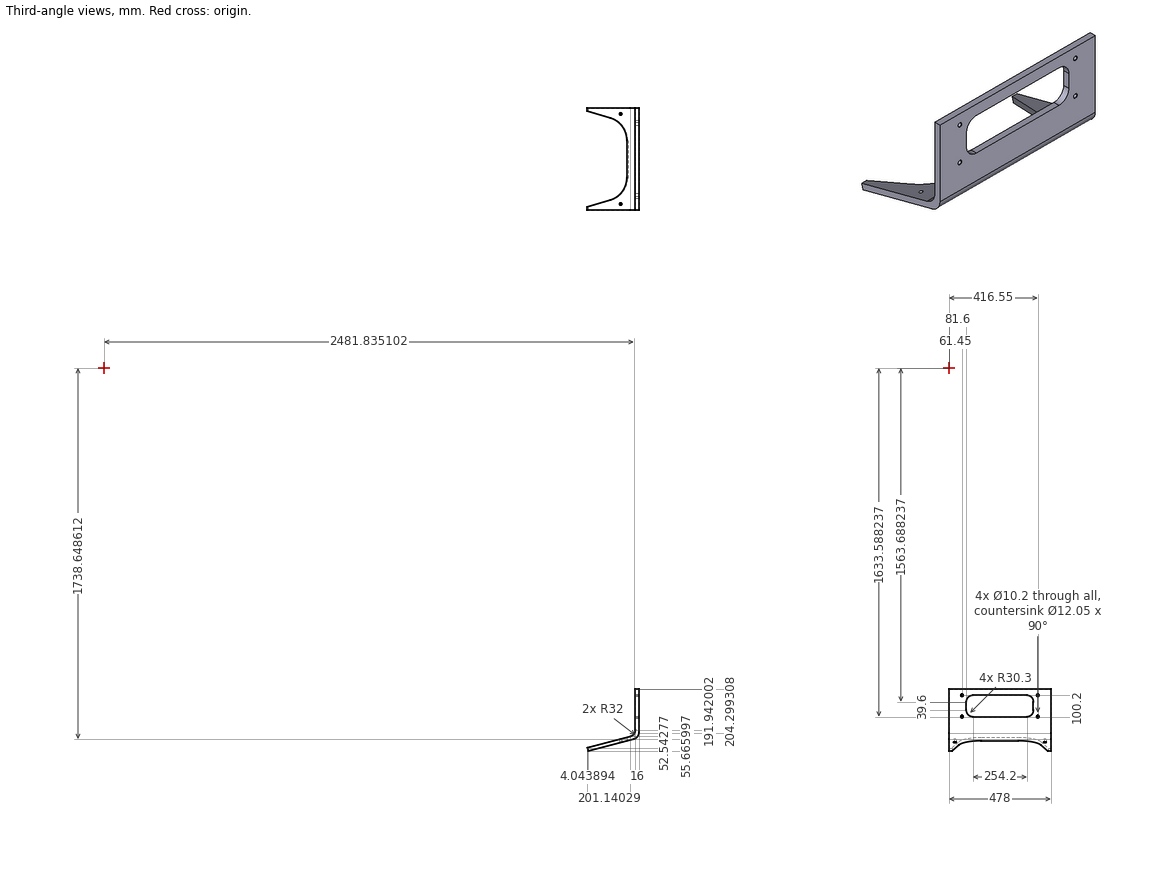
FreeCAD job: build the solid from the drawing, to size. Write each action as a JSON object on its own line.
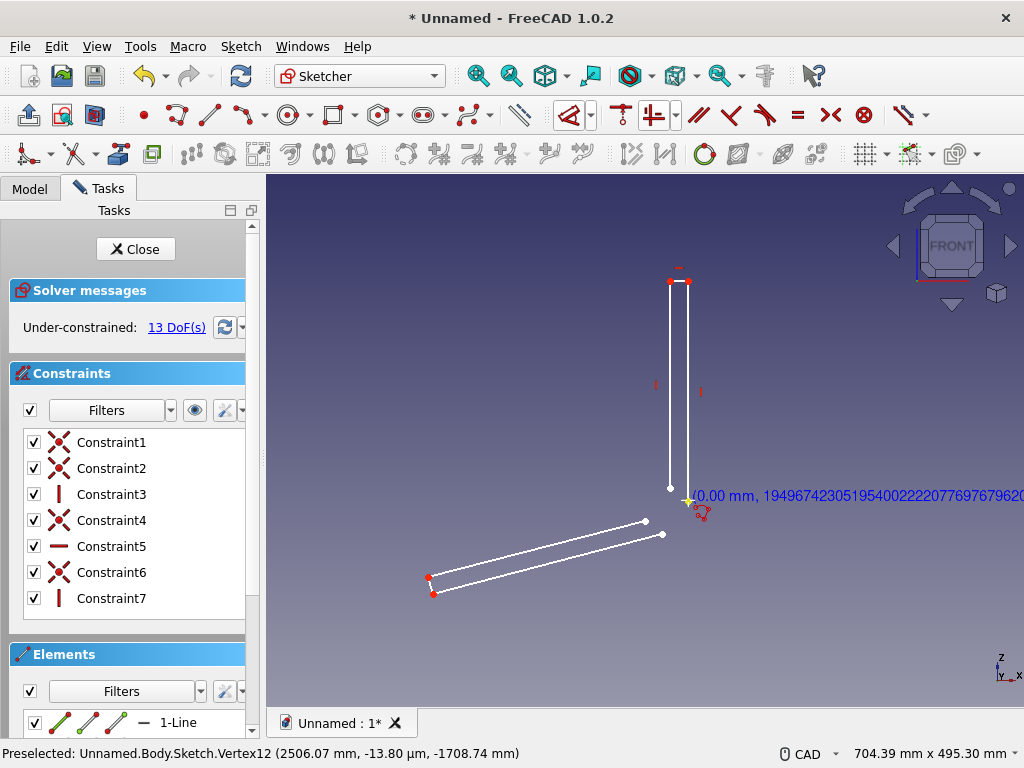
{"action": "left_click", "coordinate": [242, 116]}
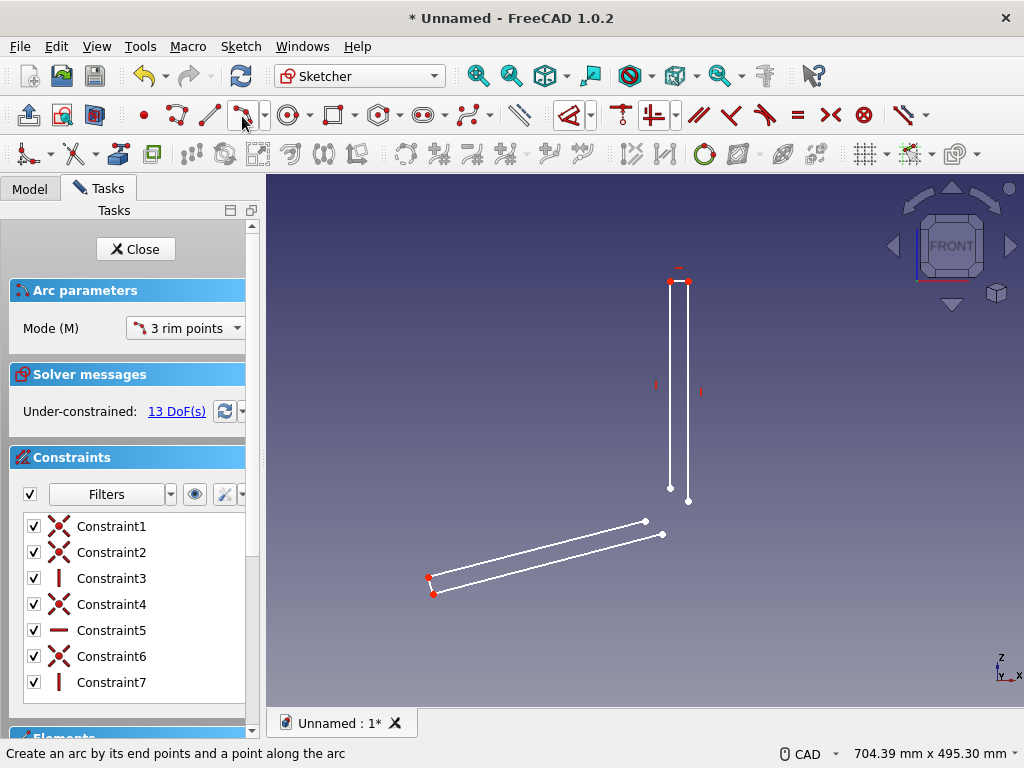
{"action": "left_click", "coordinate": [645, 521]}
{"action": "left_click", "coordinate": [670, 488]}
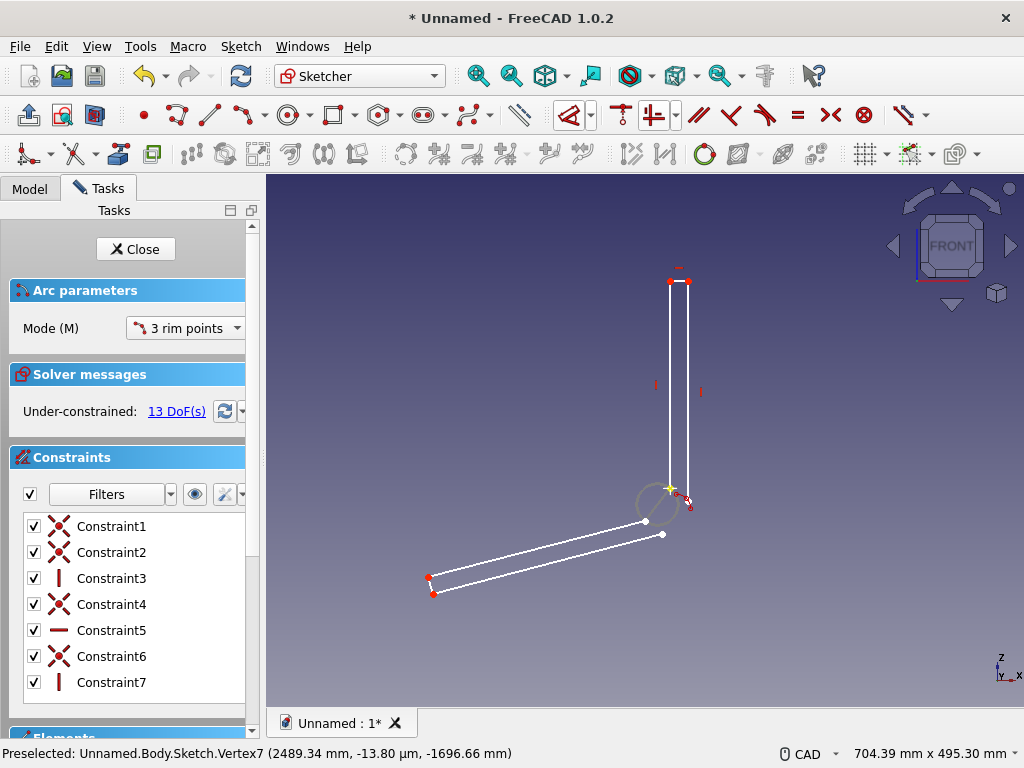
{"action": "scroll", "coordinate": [663, 508], "scroll_direction": "up", "scroll_amount": 4}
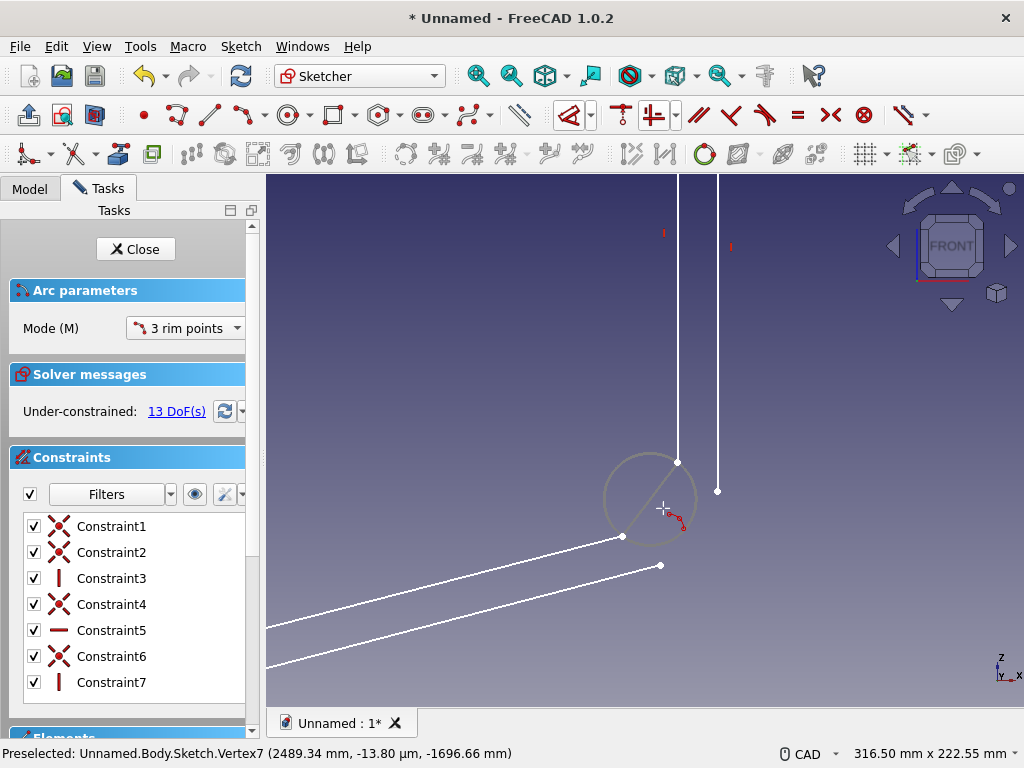
{"action": "left_click", "coordinate": [663, 506]}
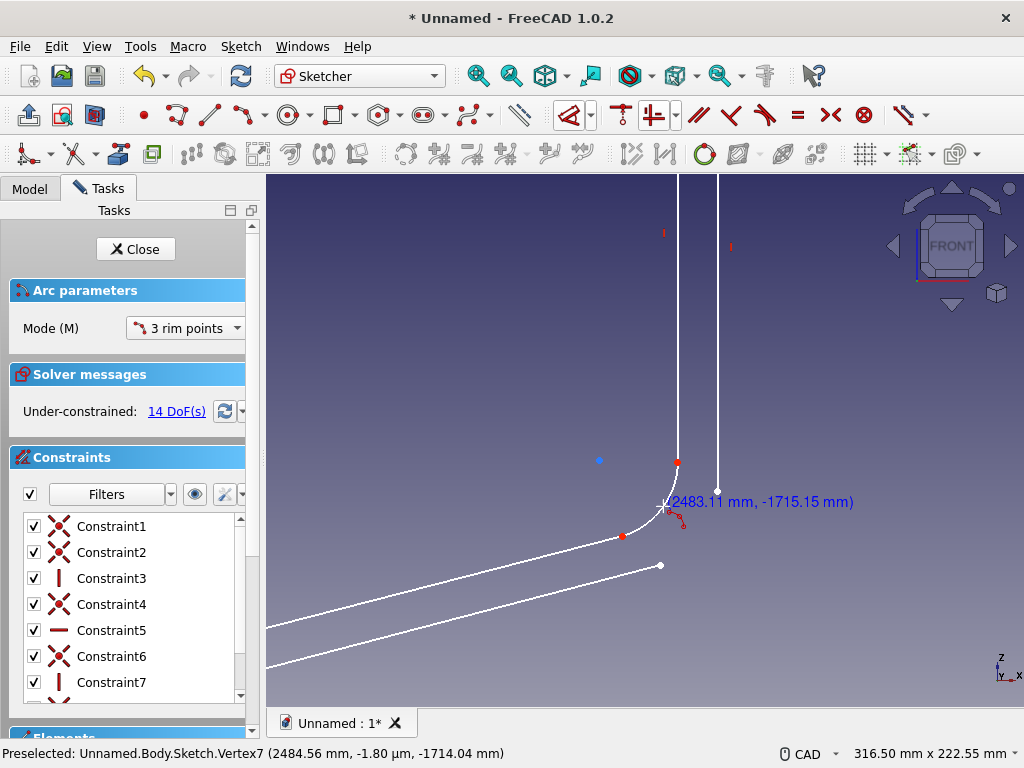
{"action": "left_click", "coordinate": [718, 492]}
{"action": "left_click", "coordinate": [660, 565]}
{"action": "left_click", "coordinate": [701, 536]}
{"action": "key", "text": "Escape"}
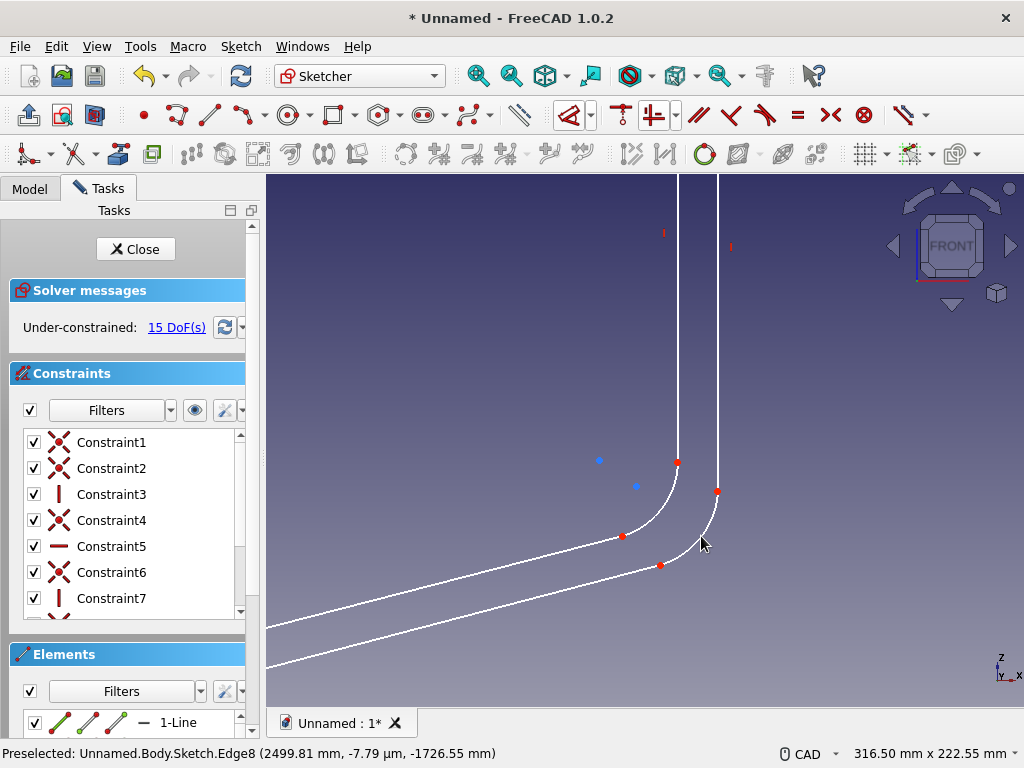
{"action": "left_click", "coordinate": [507, 605]}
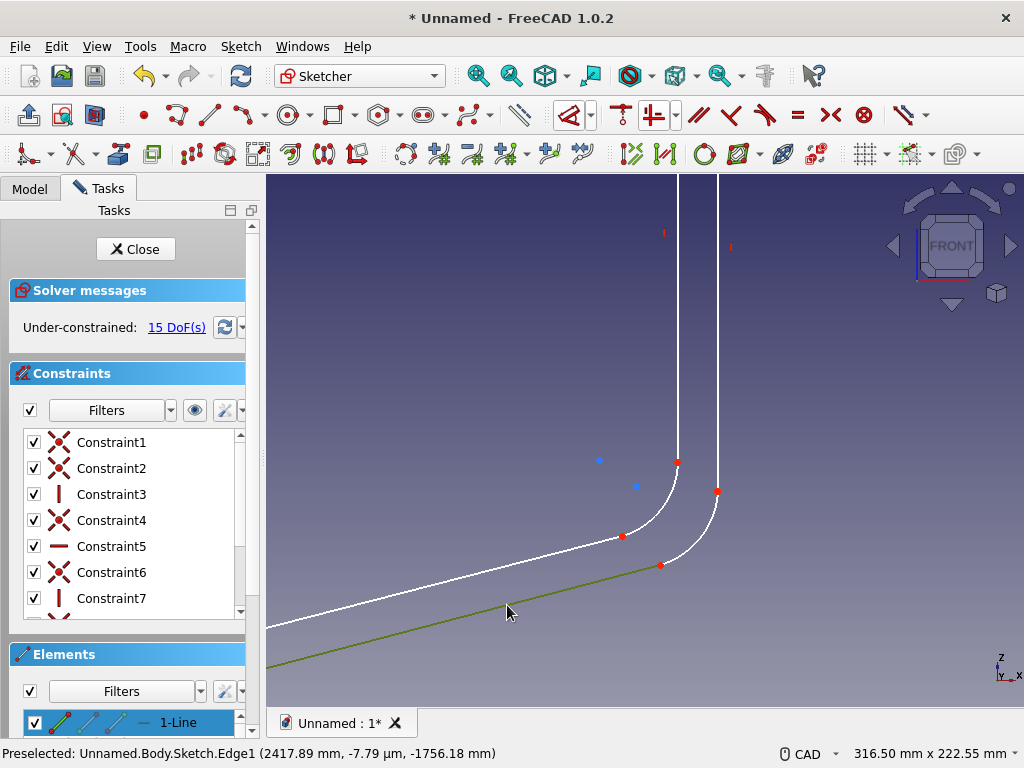
{"action": "left_click", "coordinate": [687, 551]}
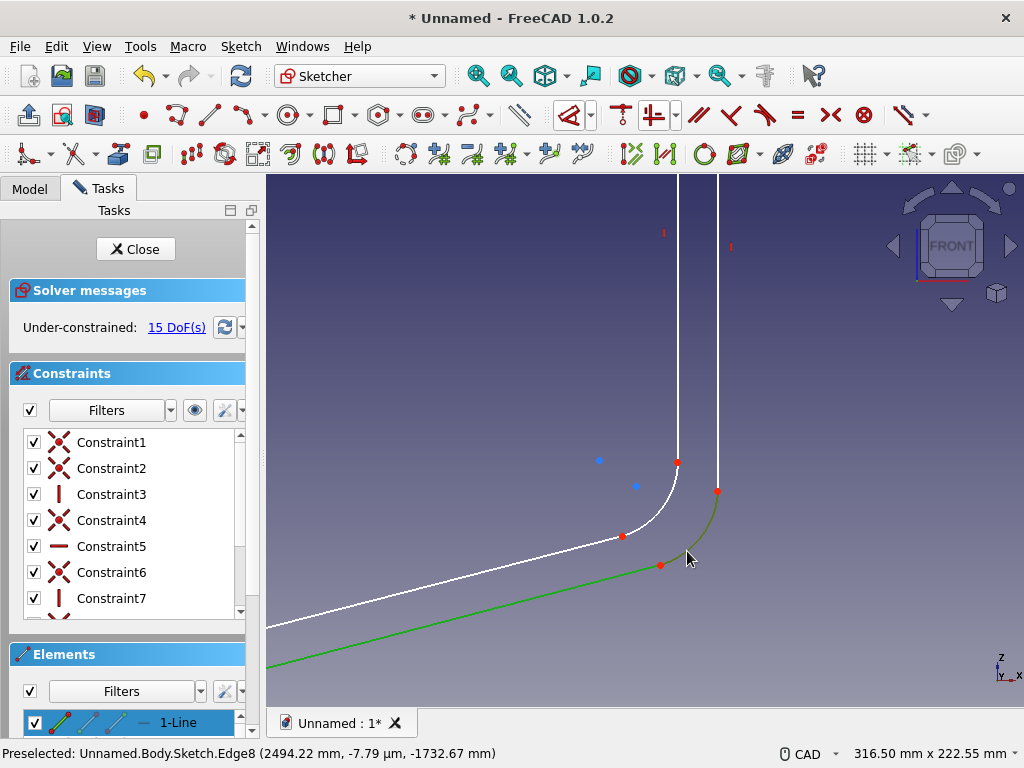
{"action": "left_click", "coordinate": [765, 116]}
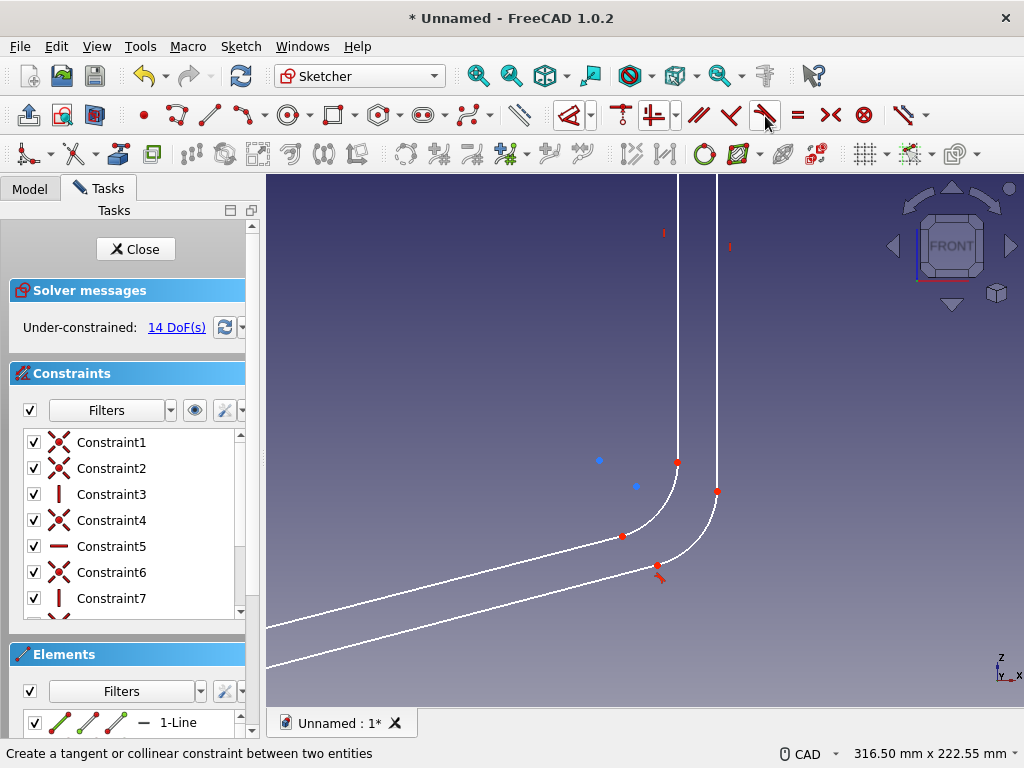
{"action": "left_click", "coordinate": [477, 574]}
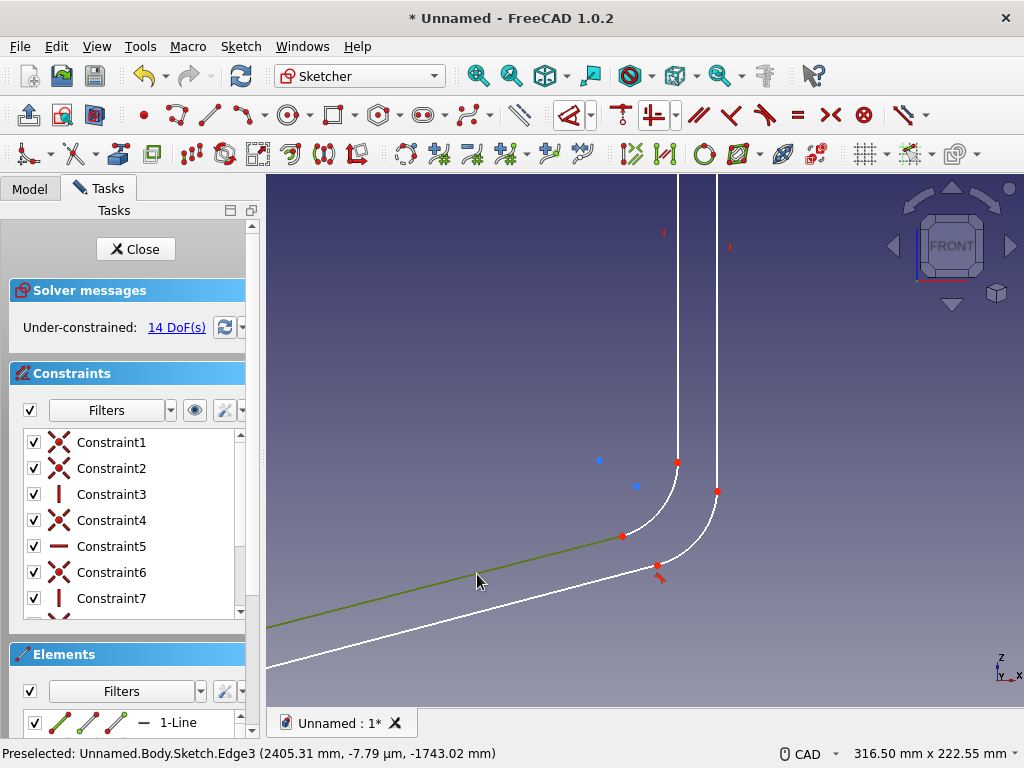
{"action": "left_click", "coordinate": [648, 522]}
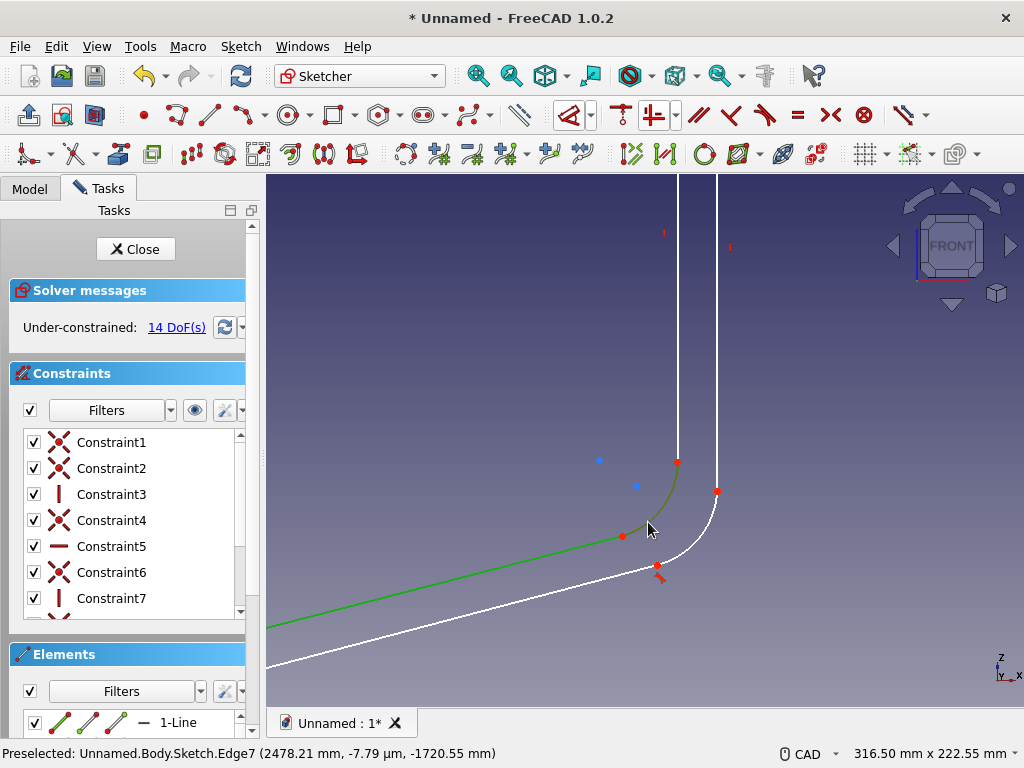
{"action": "left_click", "coordinate": [765, 116]}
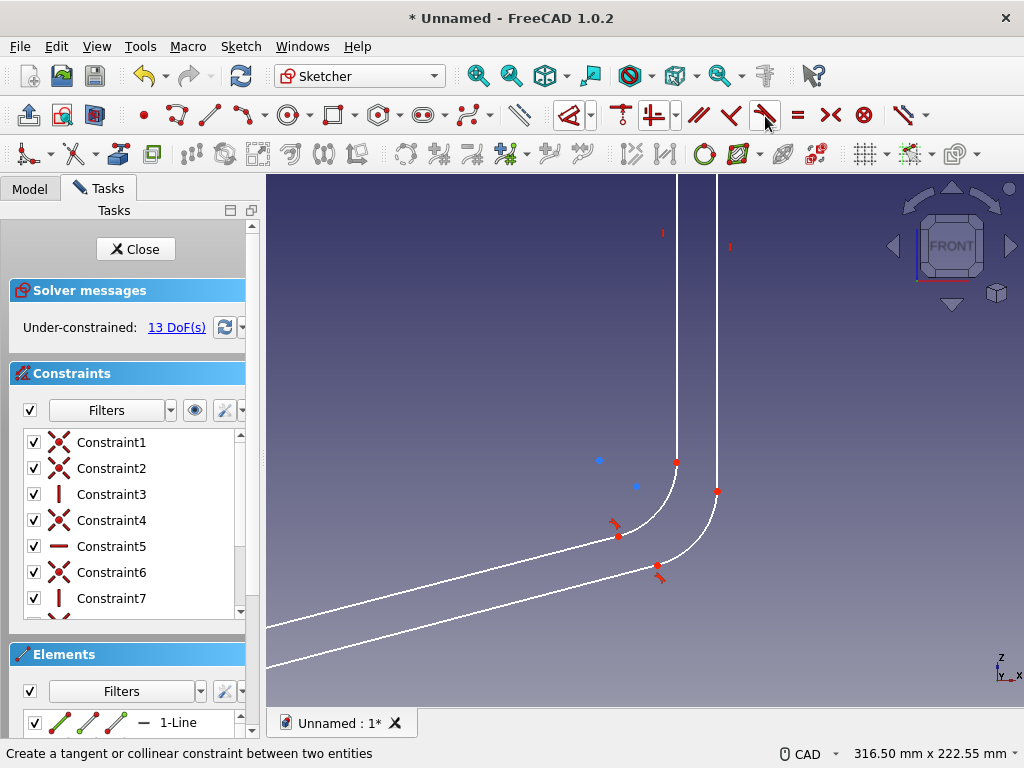
{"action": "left_click", "coordinate": [677, 325]}